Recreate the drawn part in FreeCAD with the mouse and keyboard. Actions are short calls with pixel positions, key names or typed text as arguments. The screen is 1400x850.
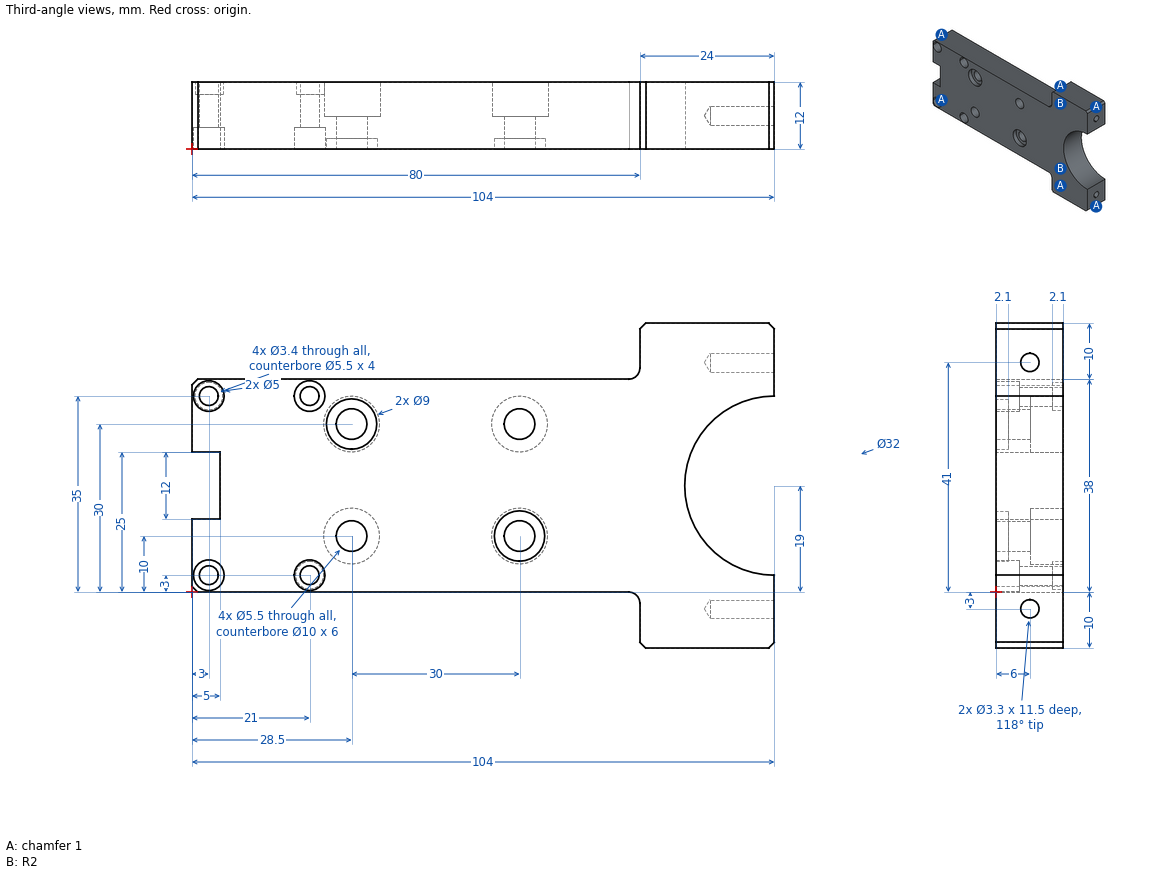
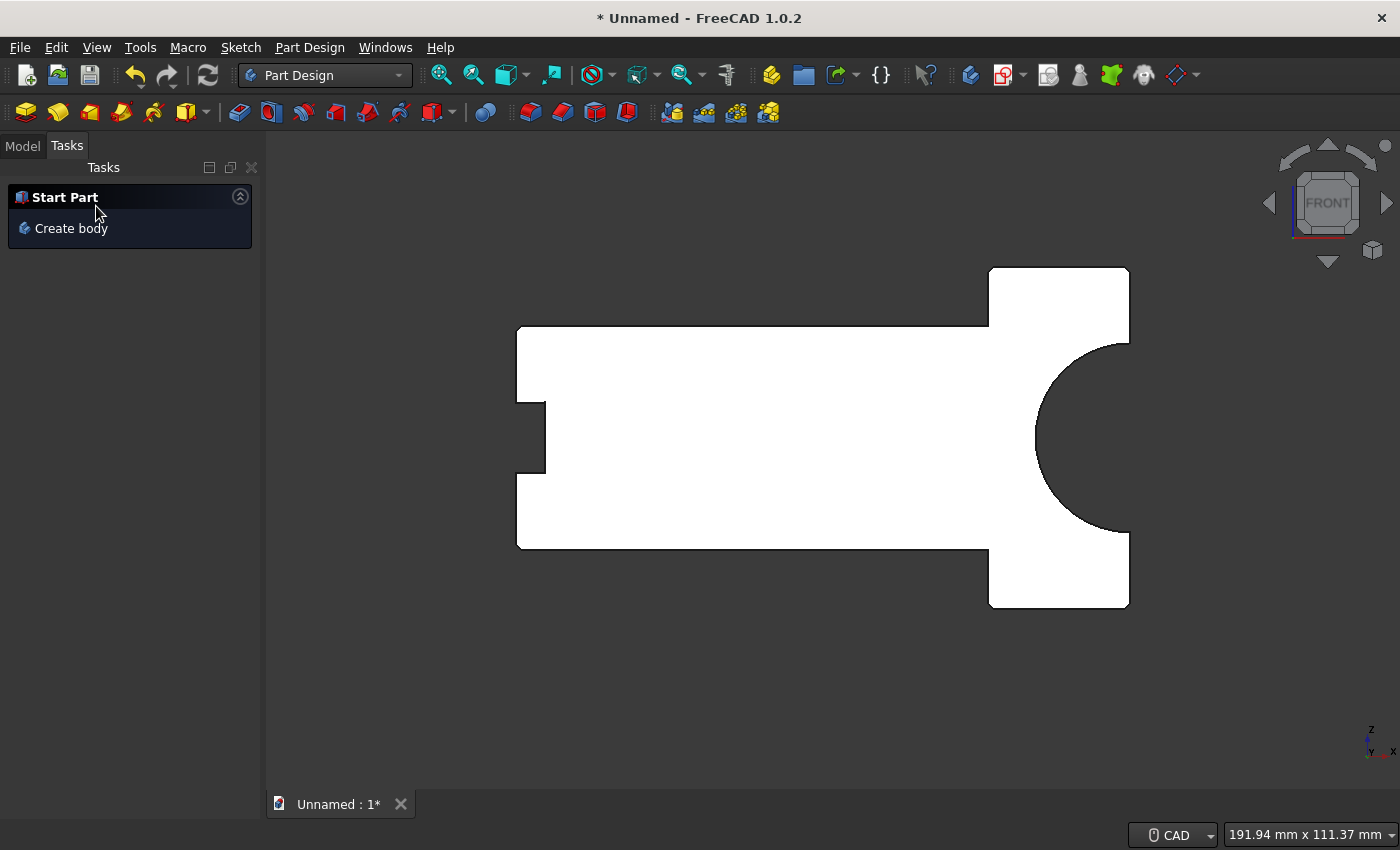
key(3)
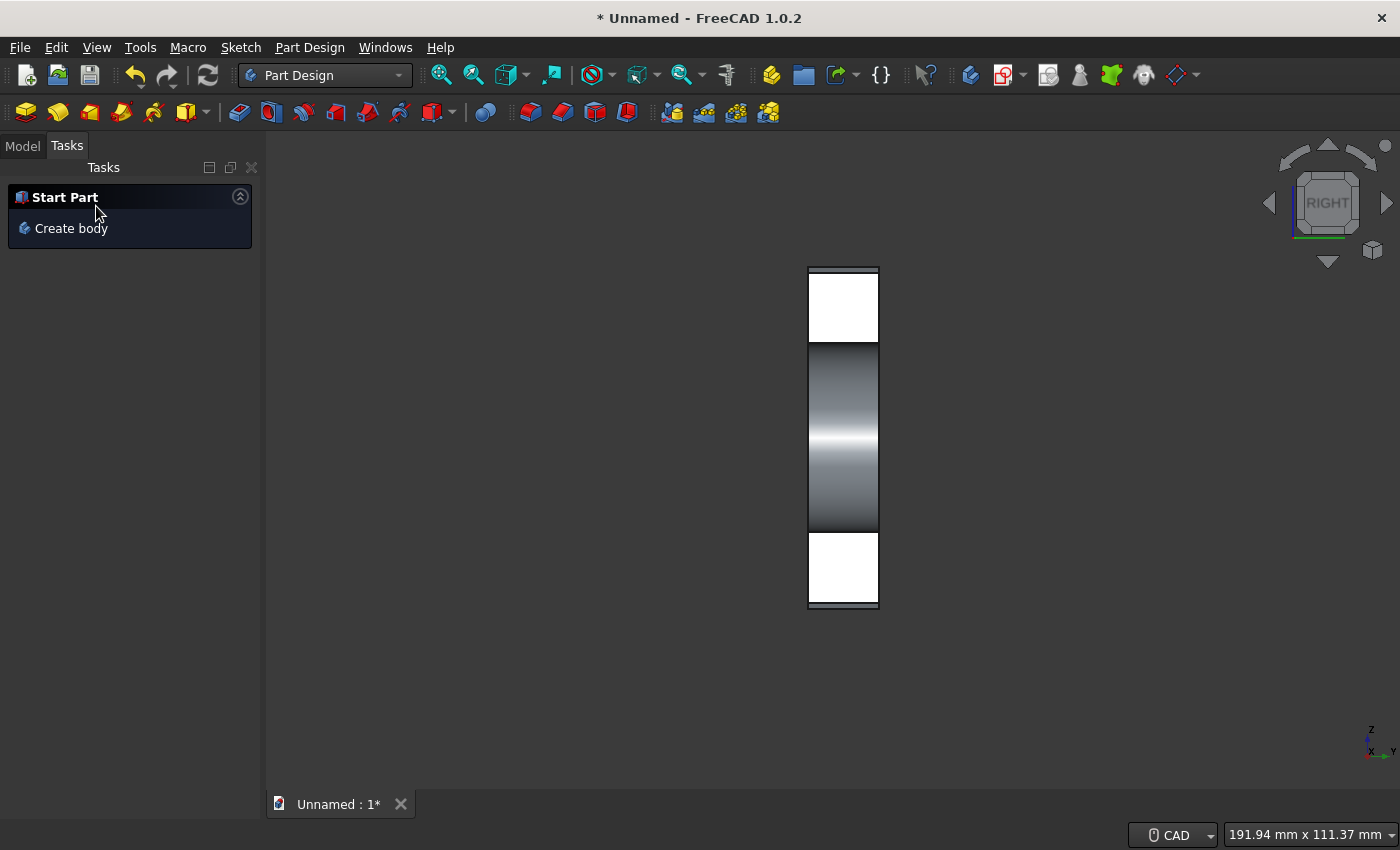
key(5)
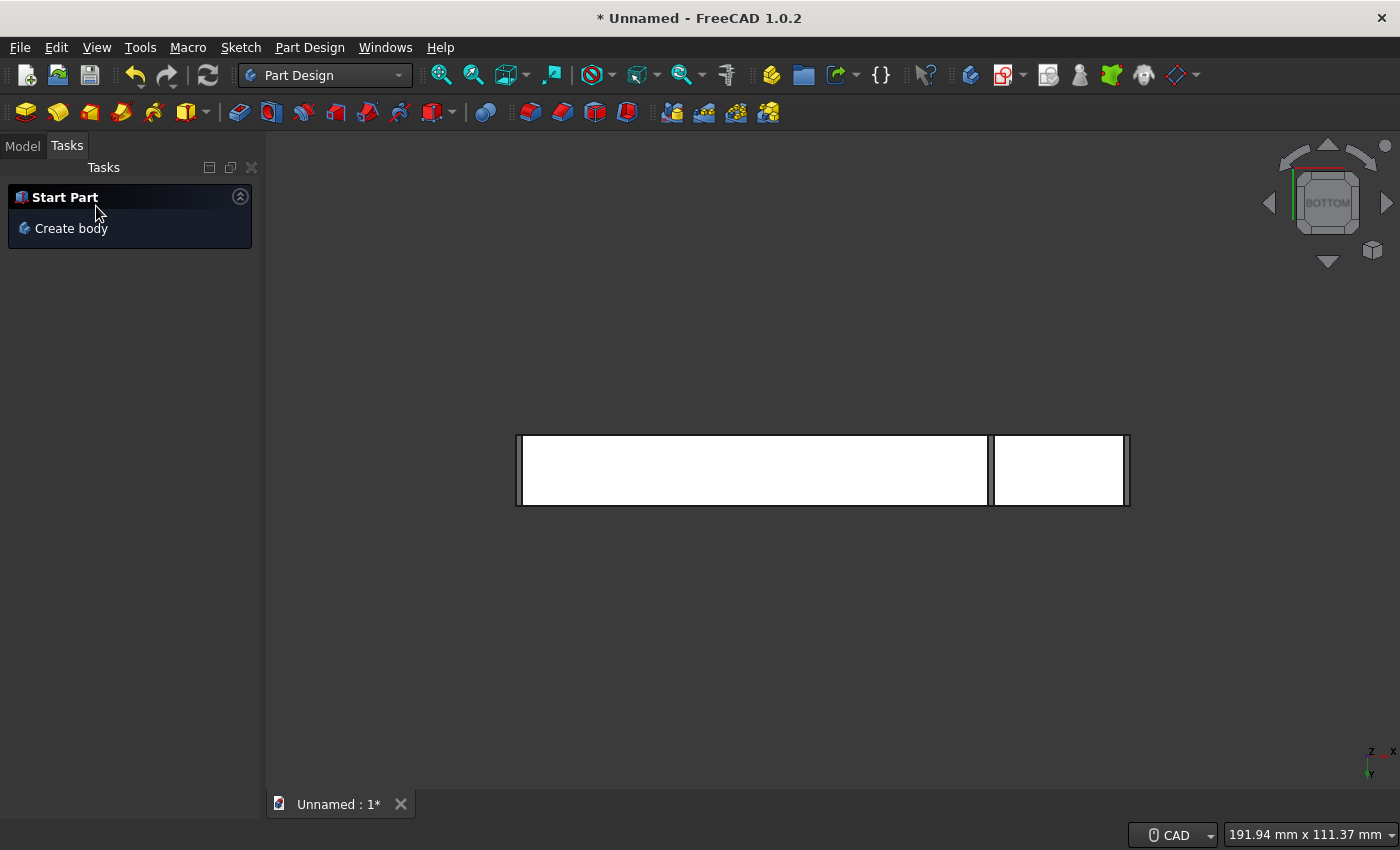
key(4)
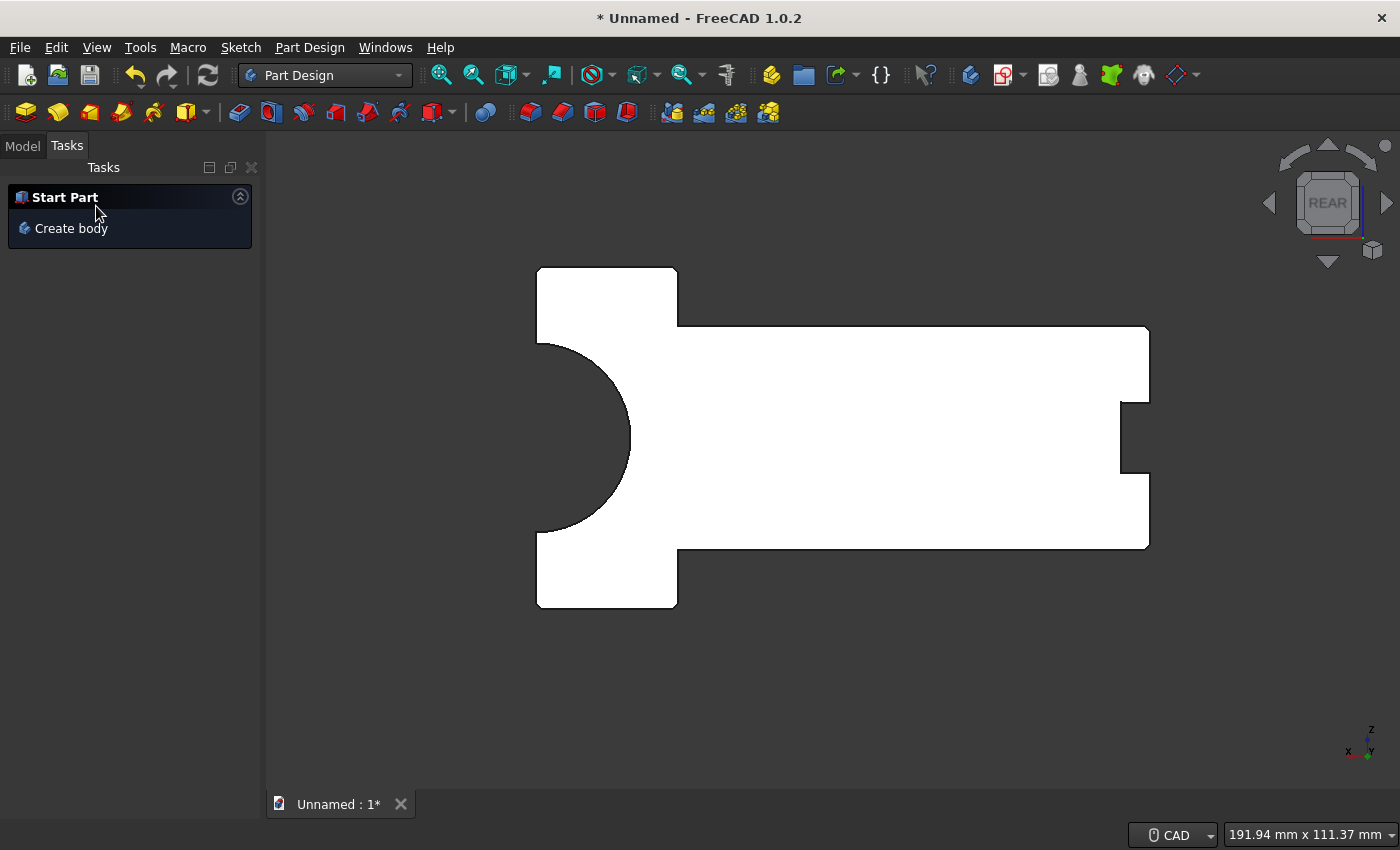
key(6)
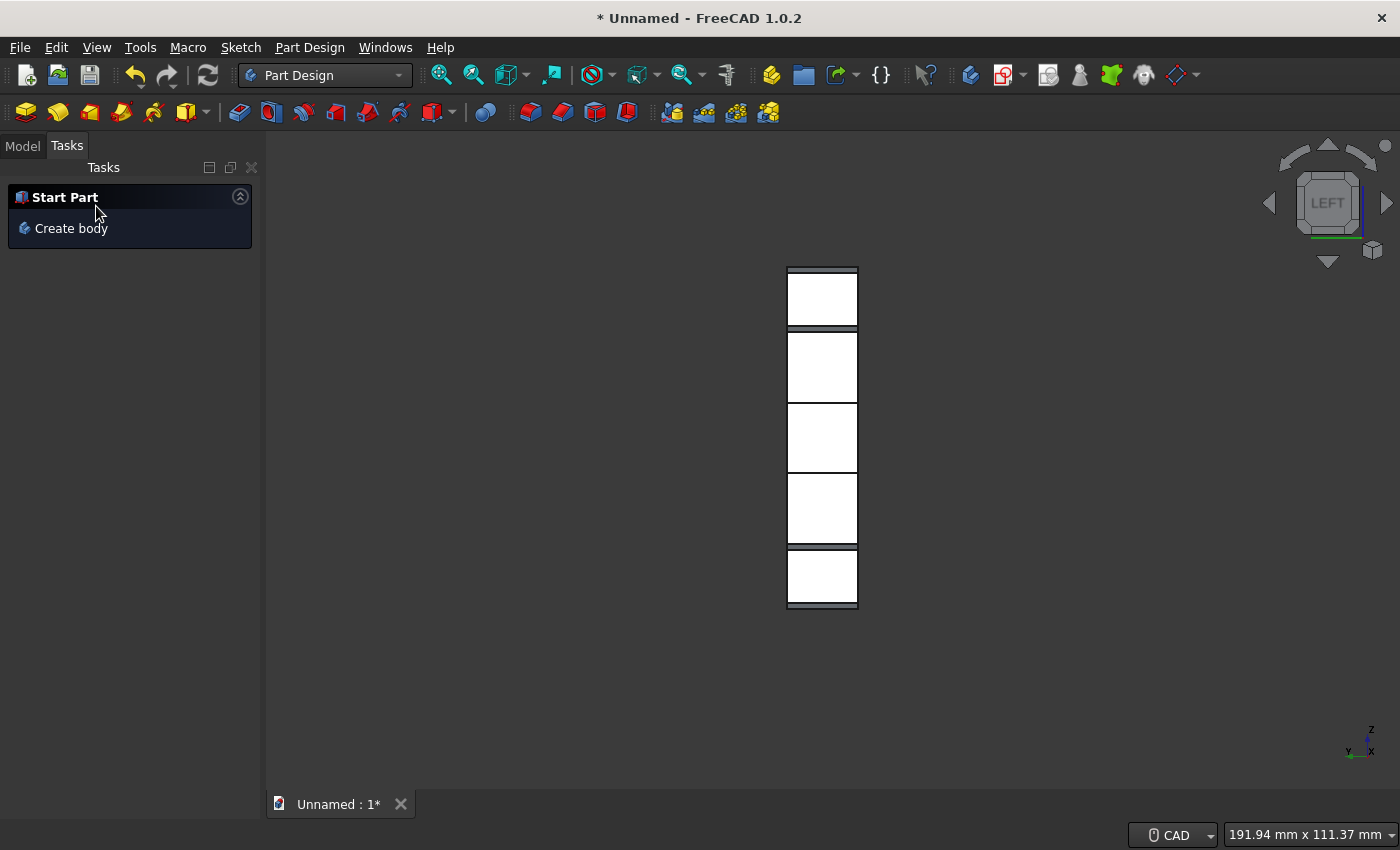
key(v)
key(3)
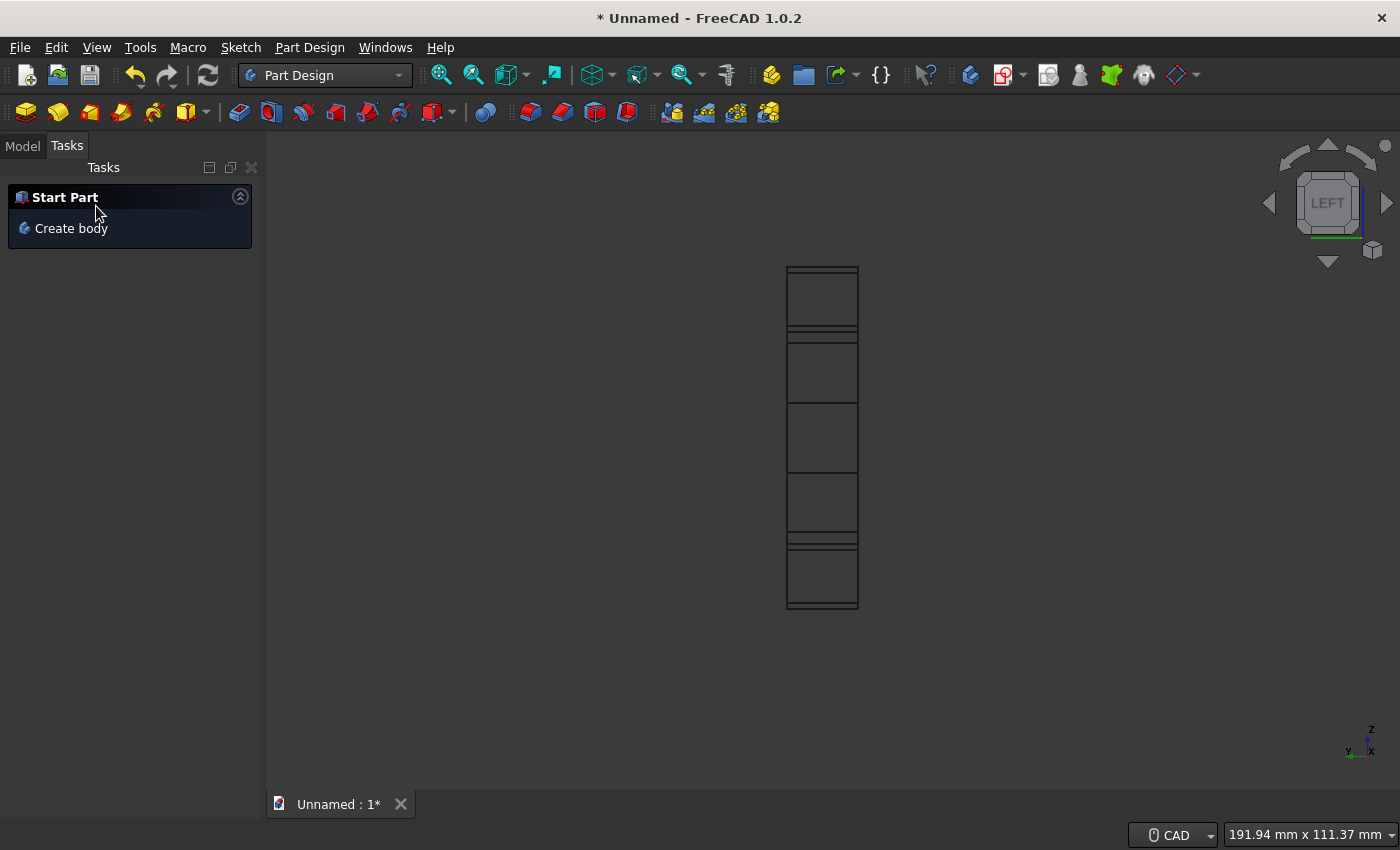
key(0)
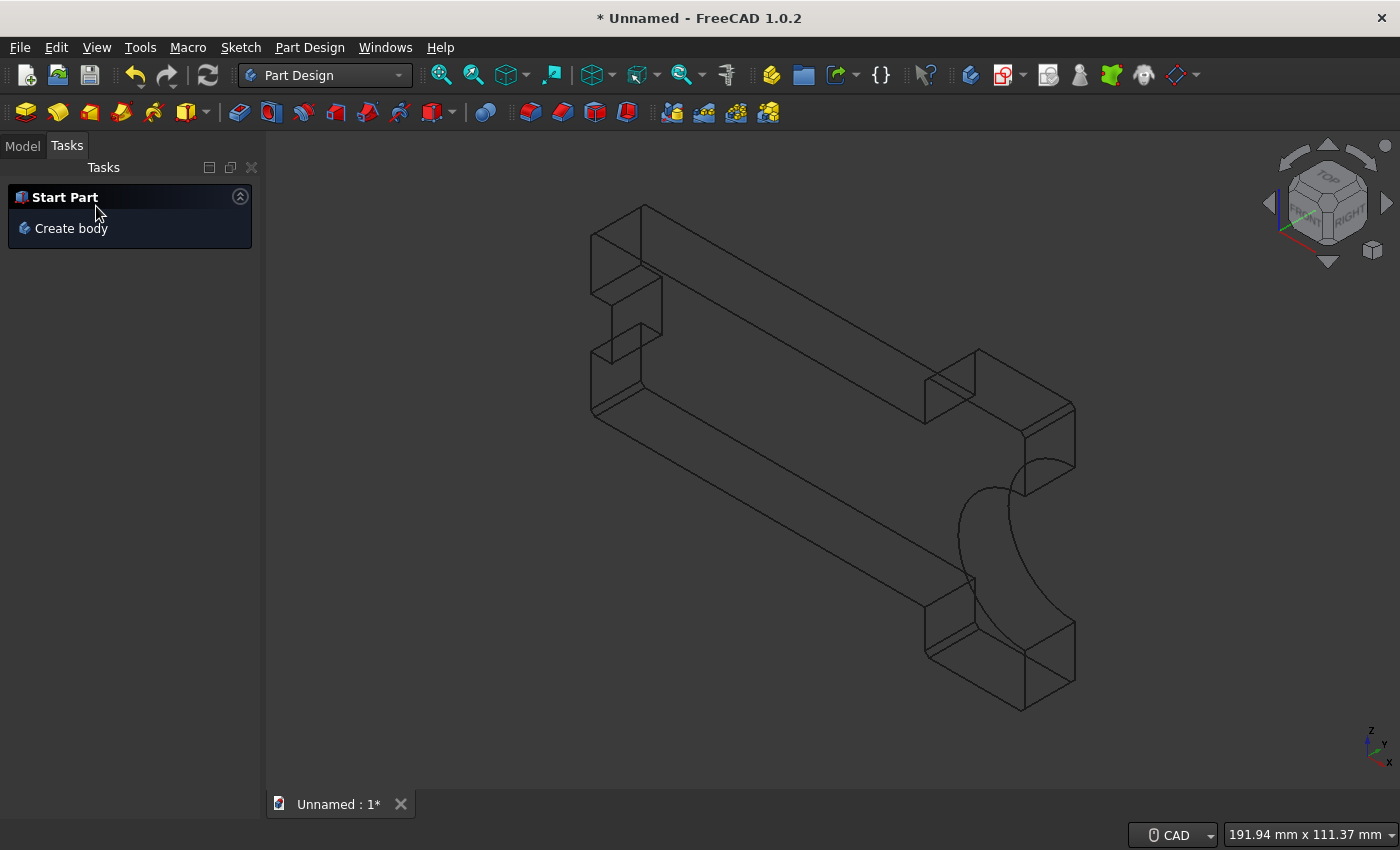
click(950, 409)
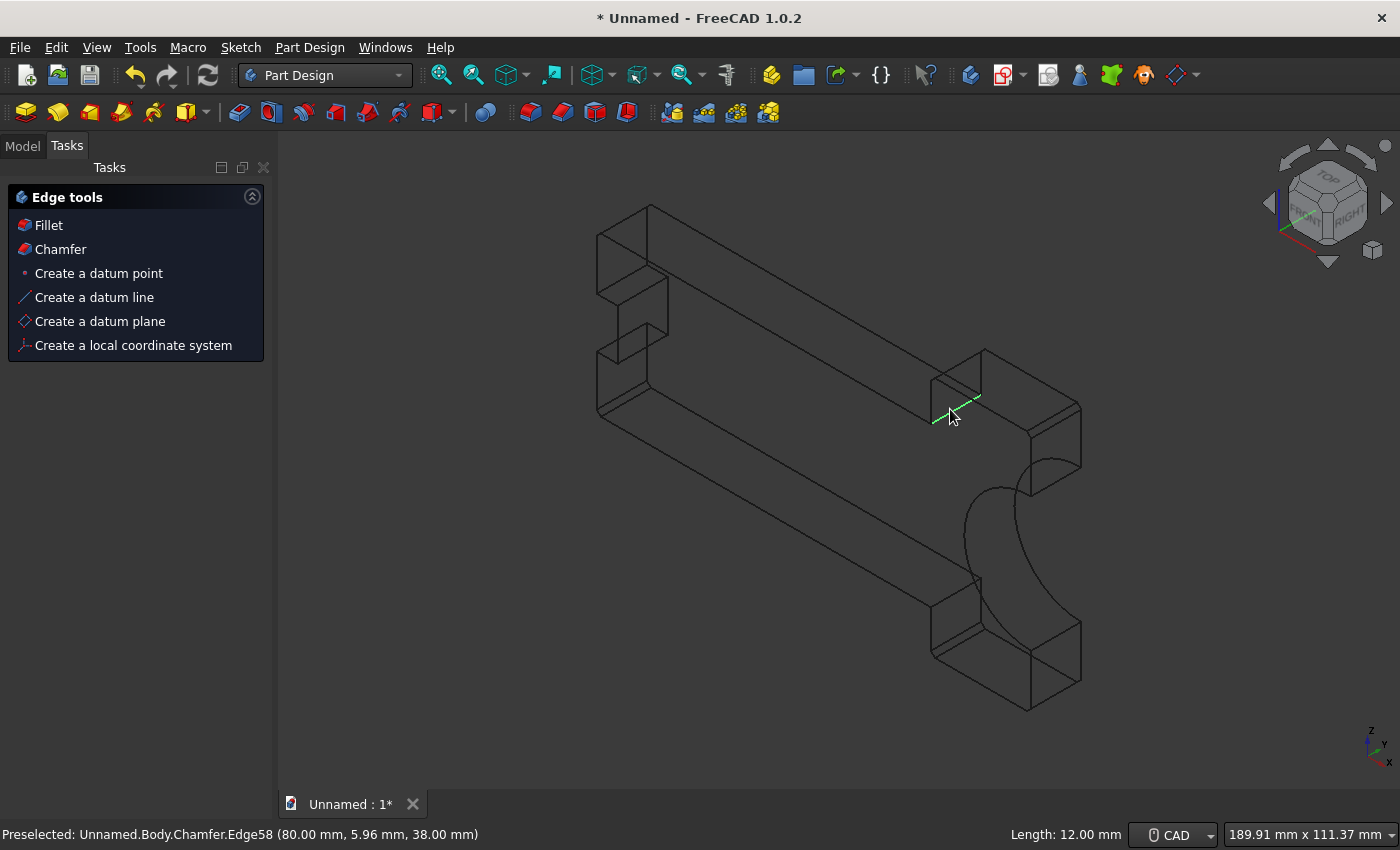
click(956, 592, ctrl)